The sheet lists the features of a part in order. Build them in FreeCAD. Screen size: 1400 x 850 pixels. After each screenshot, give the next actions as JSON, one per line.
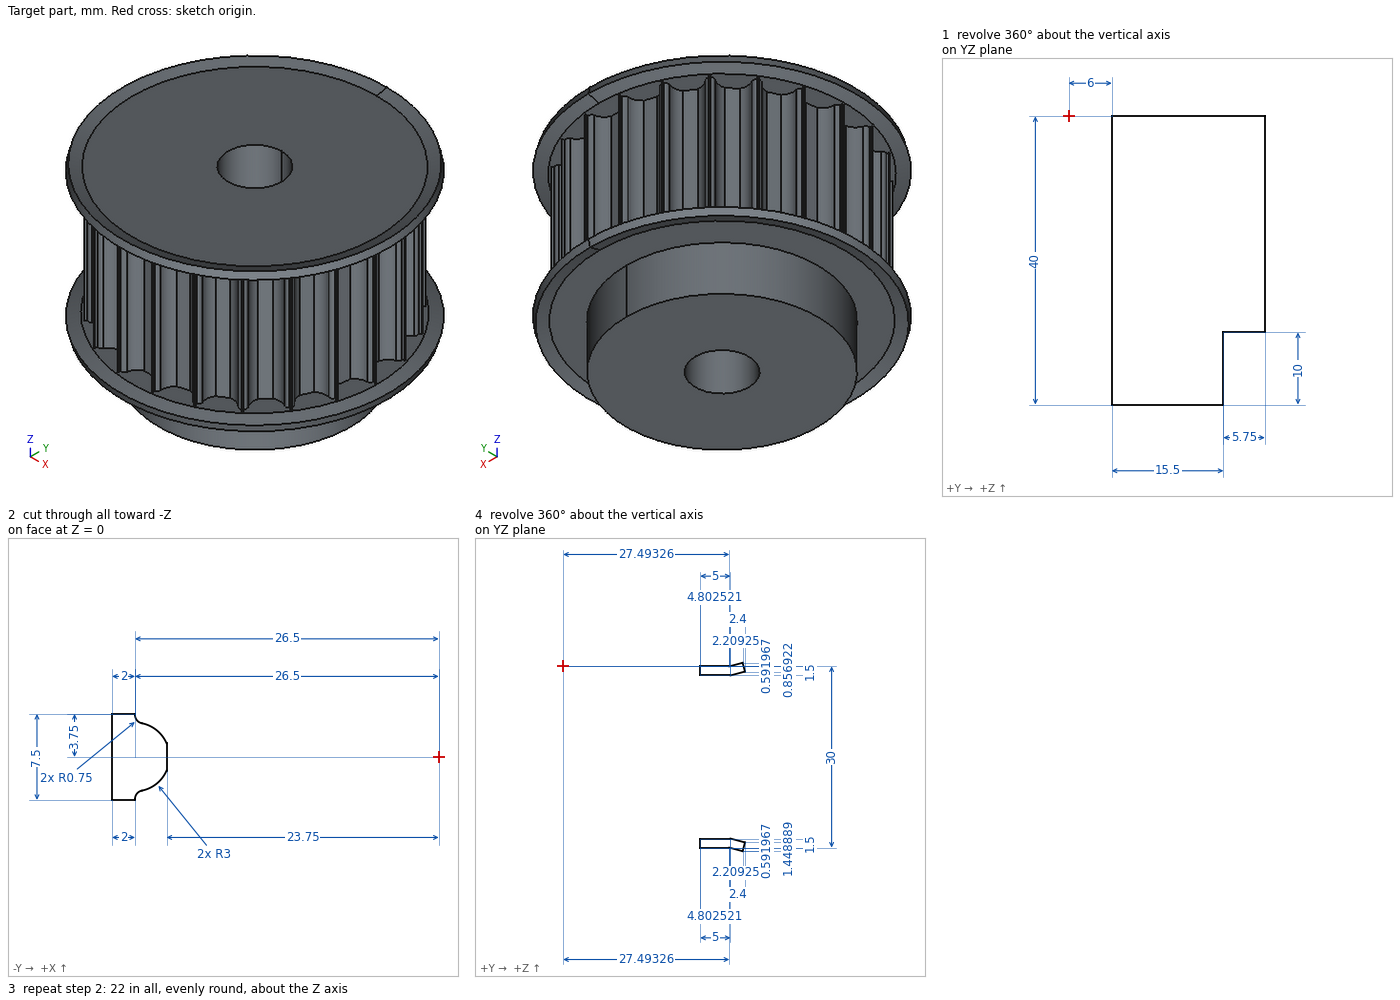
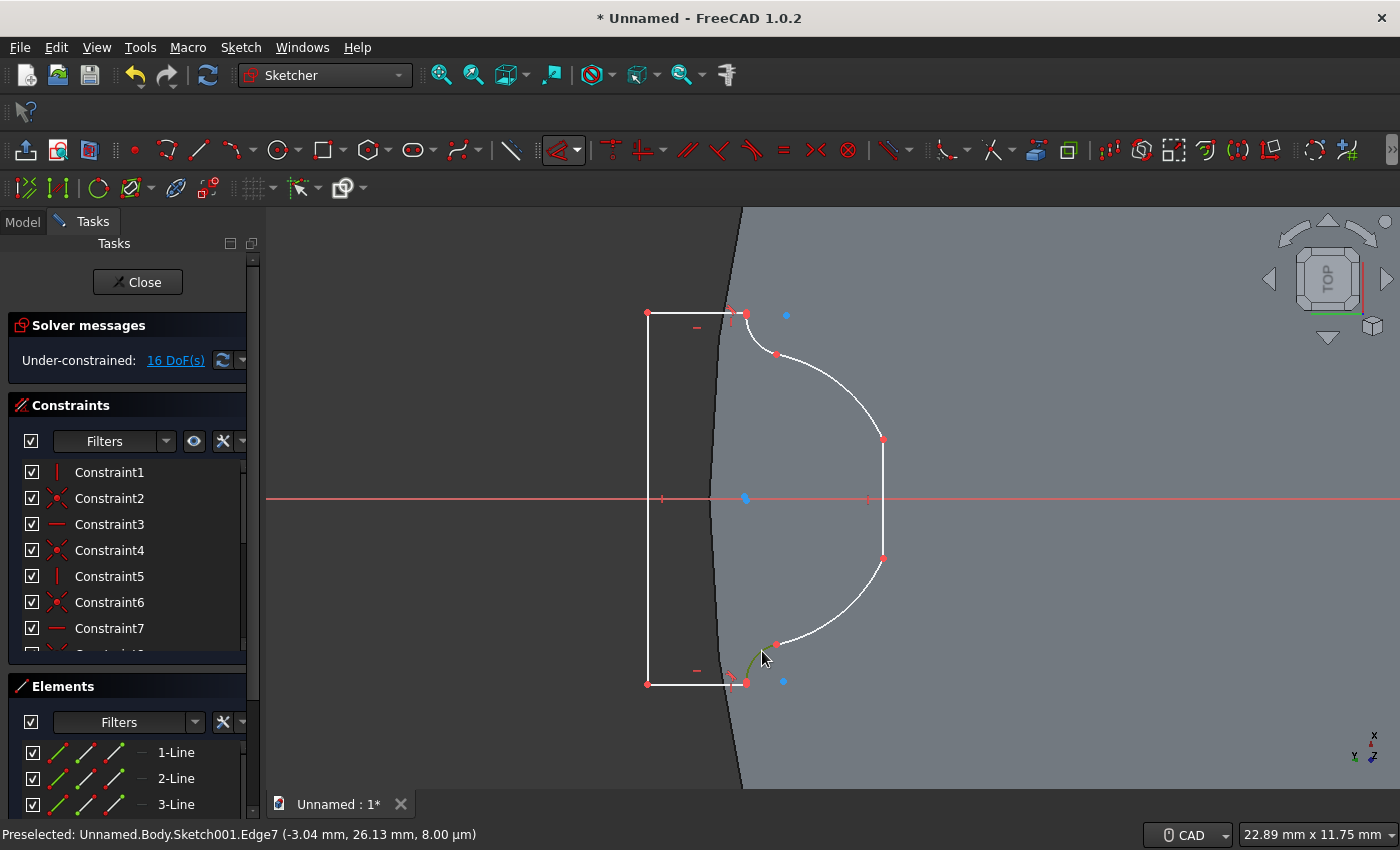
{"action": "left_click", "coordinate": [816, 630]}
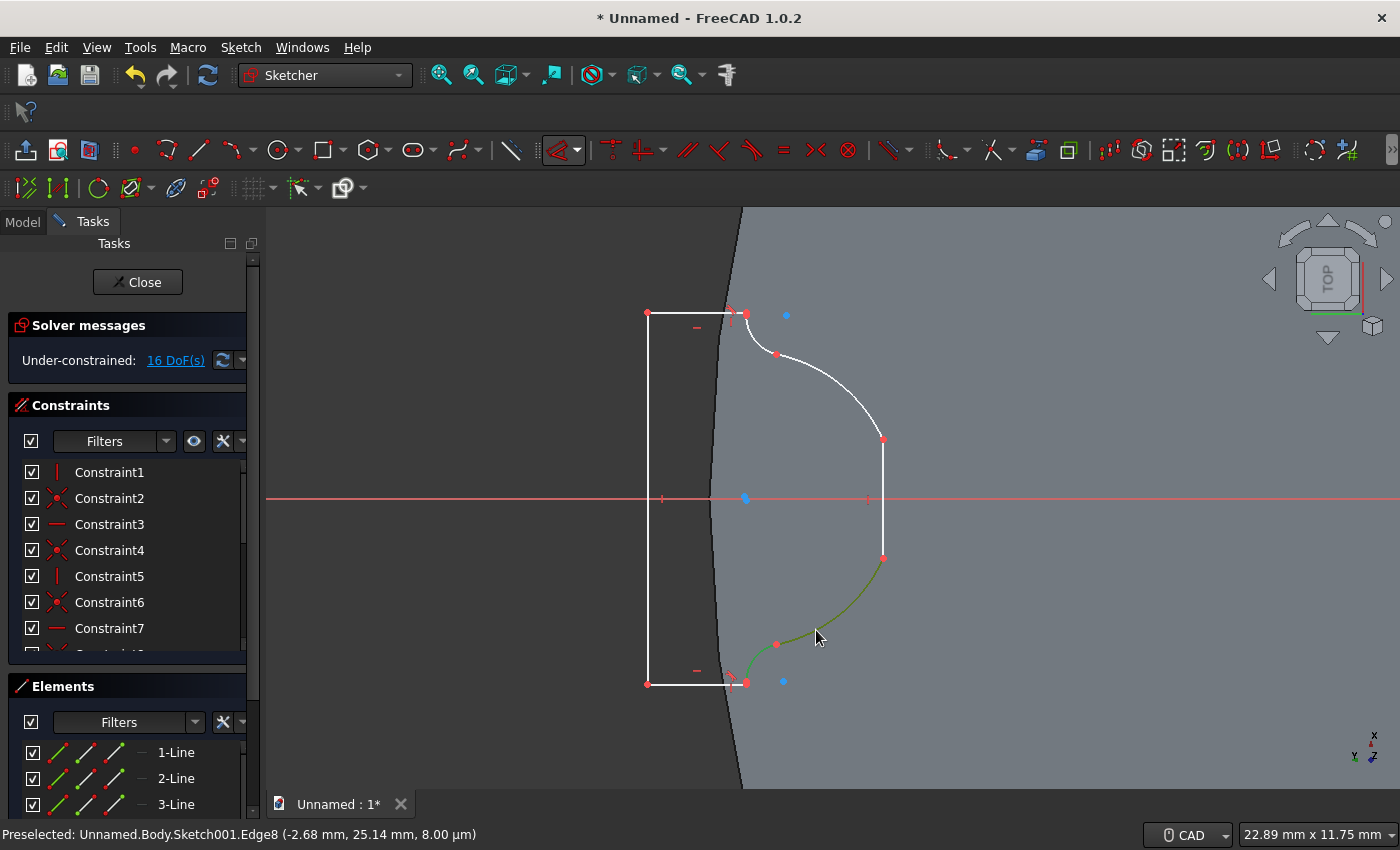
{"action": "left_click", "coordinate": [752, 150]}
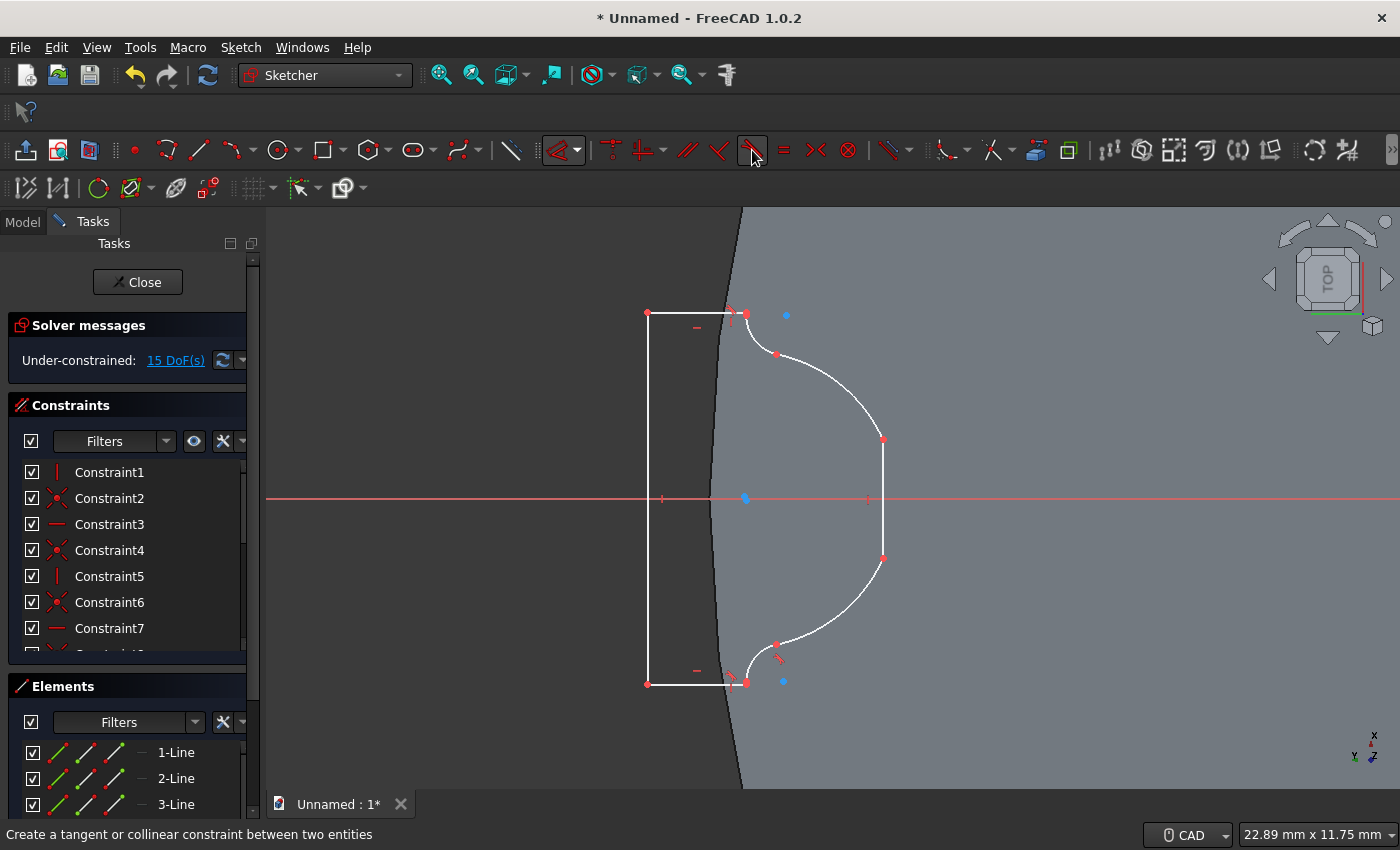
{"action": "left_click", "coordinate": [860, 404]}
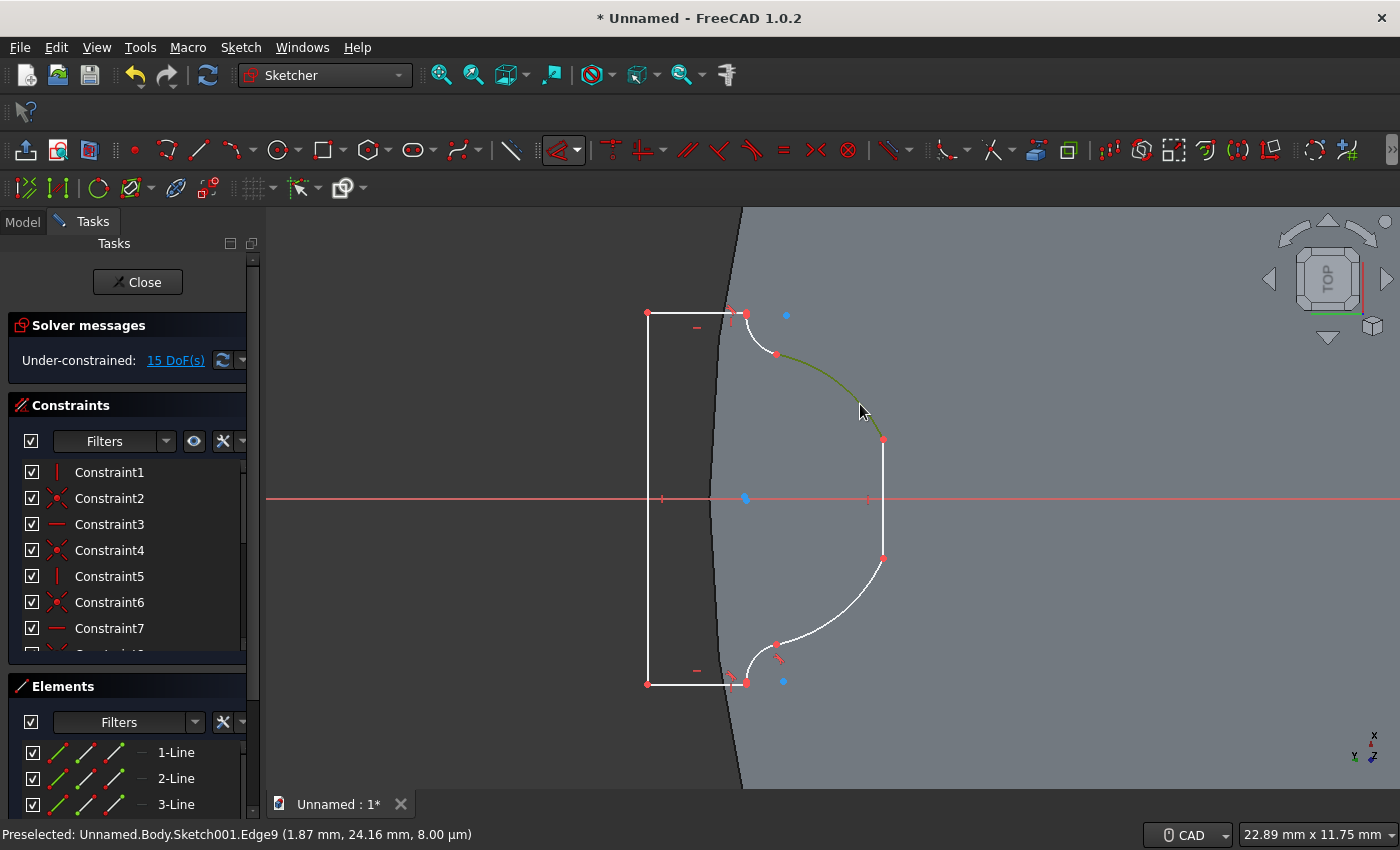
{"action": "left_click", "coordinate": [749, 331]}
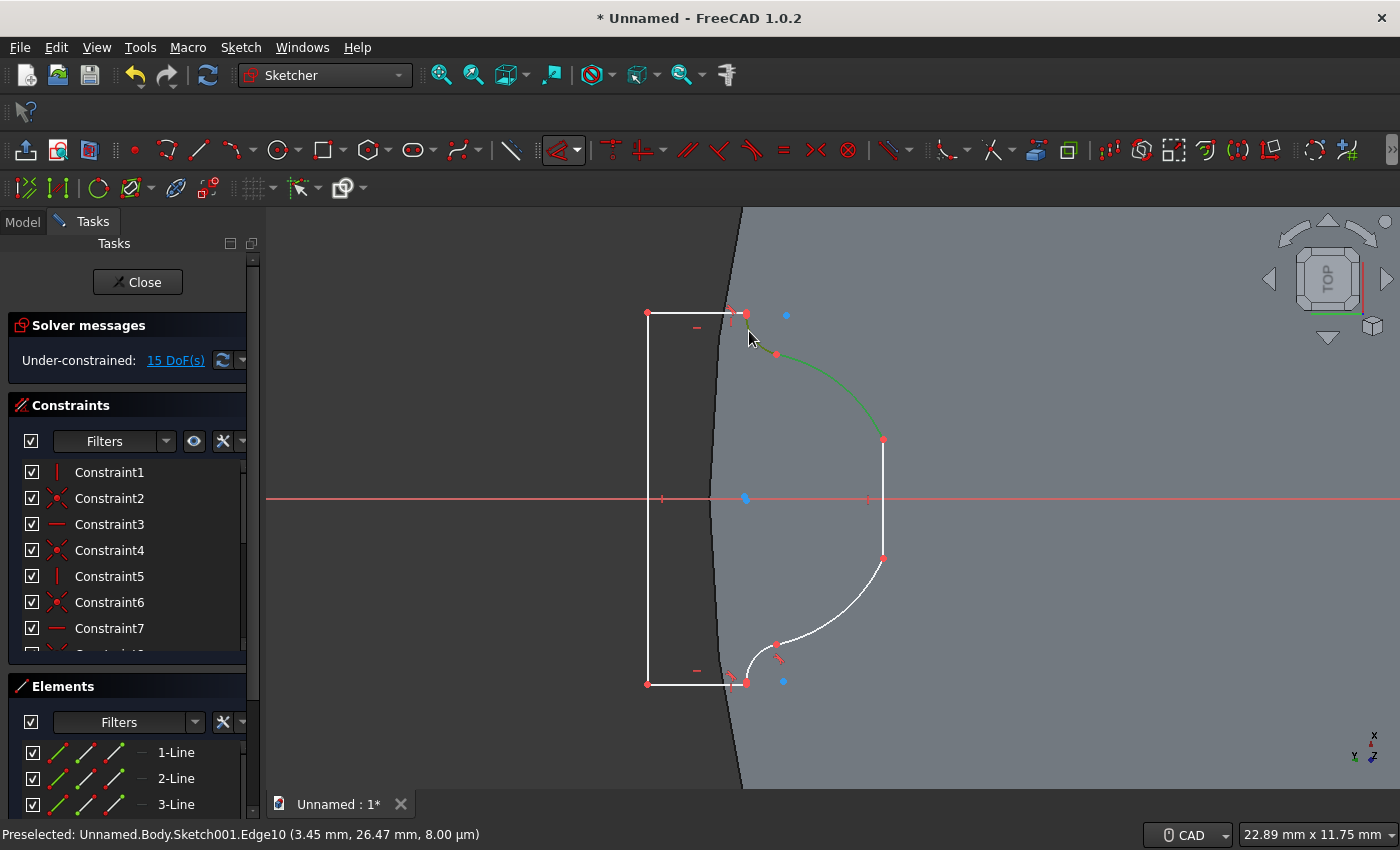
{"action": "left_click", "coordinate": [752, 150]}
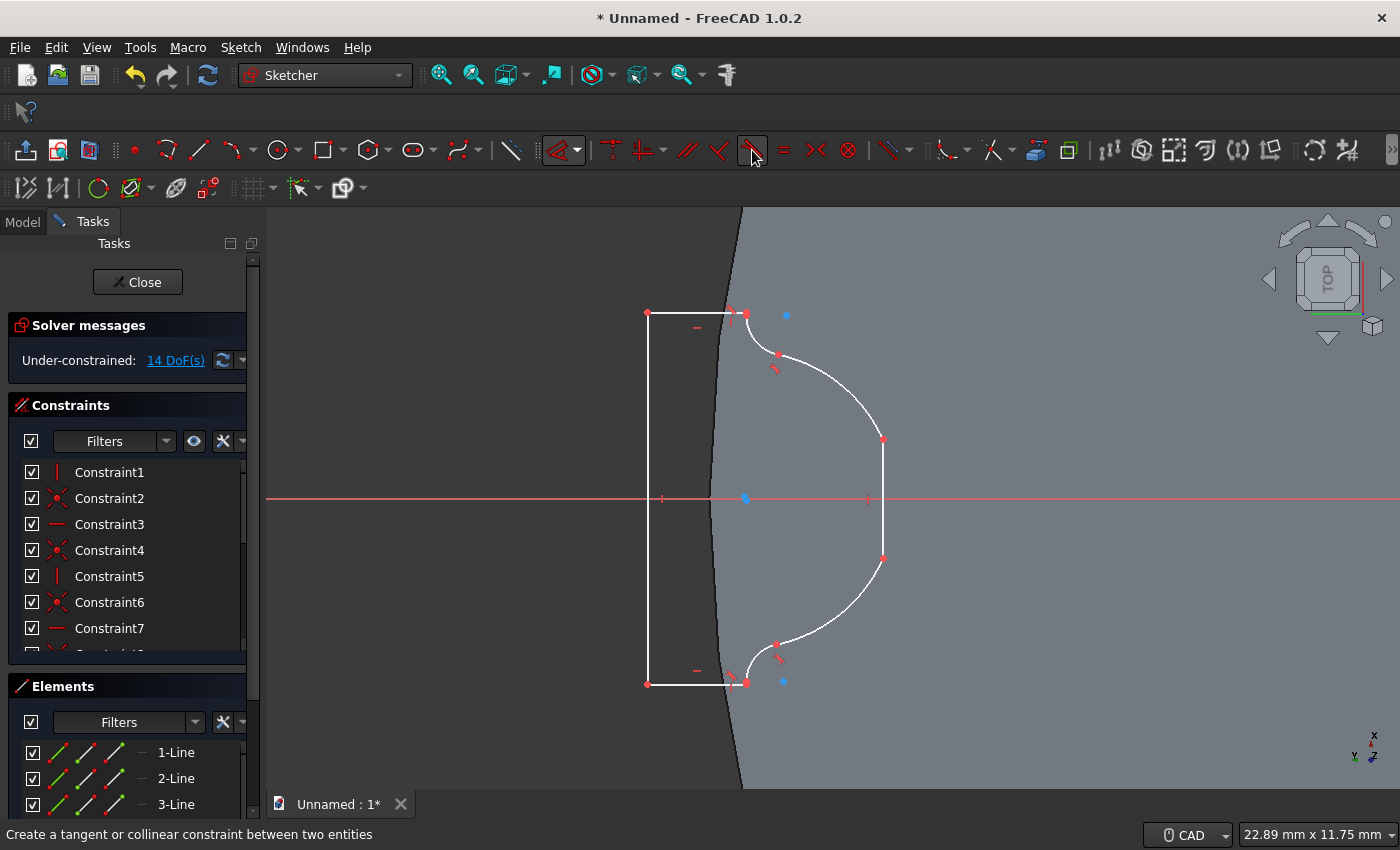
{"action": "left_click", "coordinate": [816, 630]}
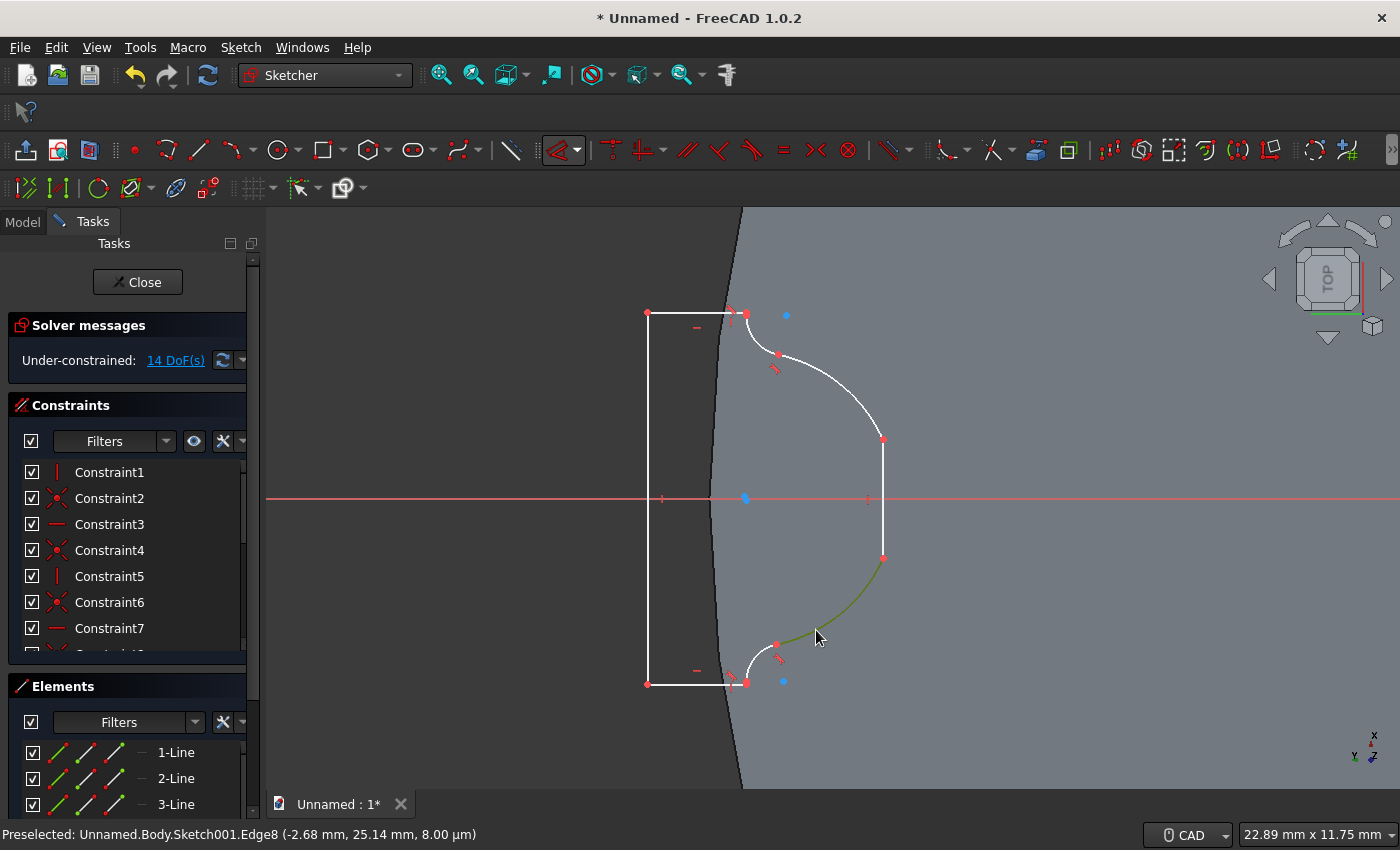
{"action": "left_click", "coordinate": [861, 404]}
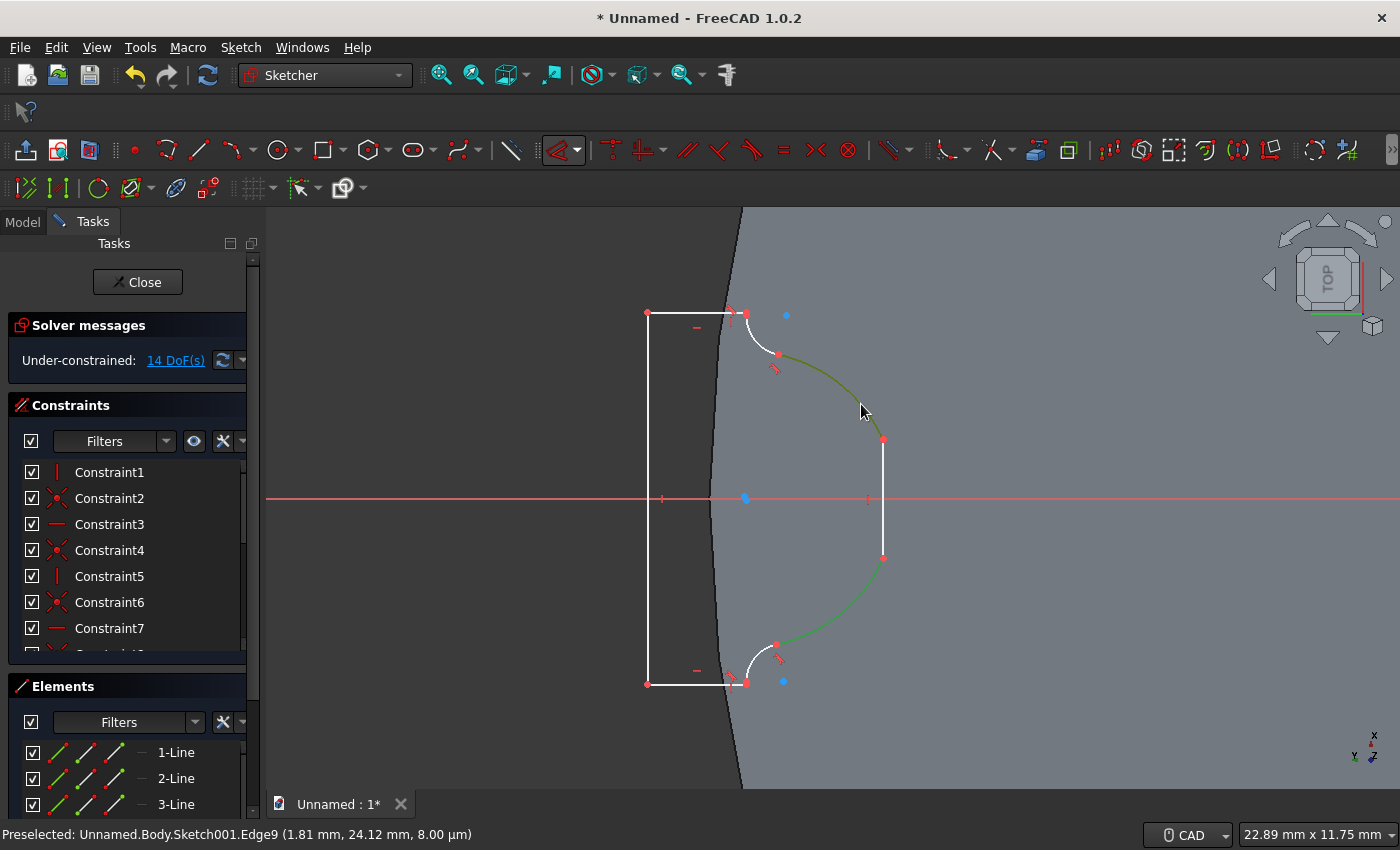
{"action": "left_click", "coordinate": [612, 150]}